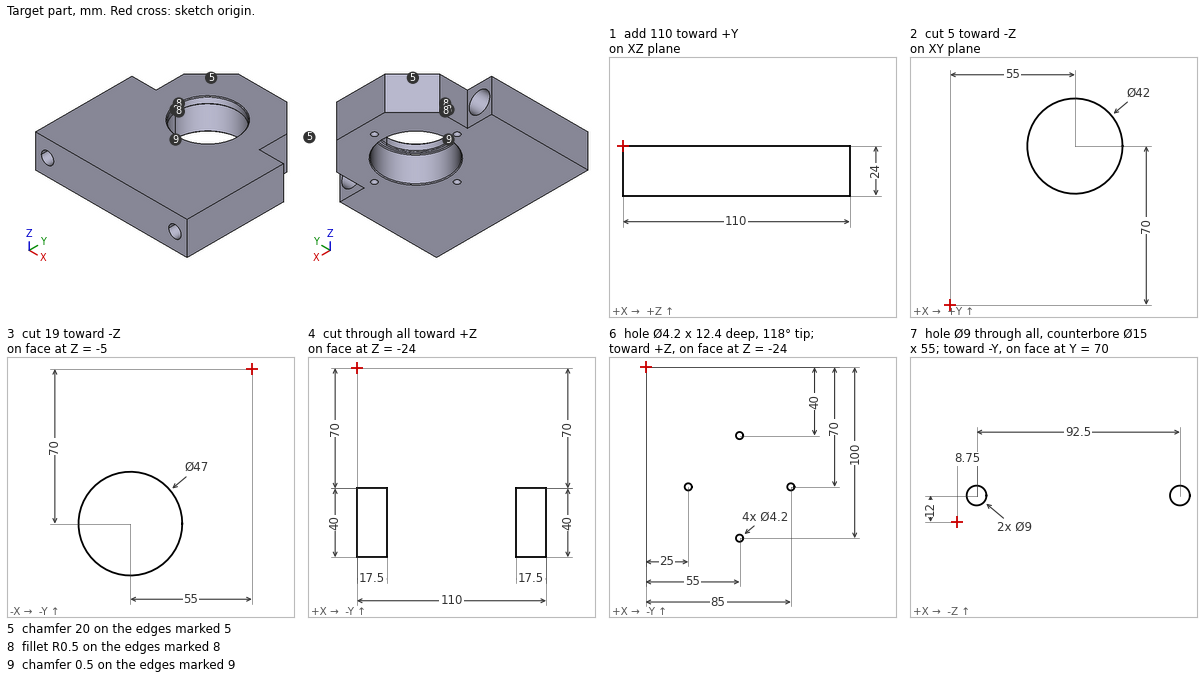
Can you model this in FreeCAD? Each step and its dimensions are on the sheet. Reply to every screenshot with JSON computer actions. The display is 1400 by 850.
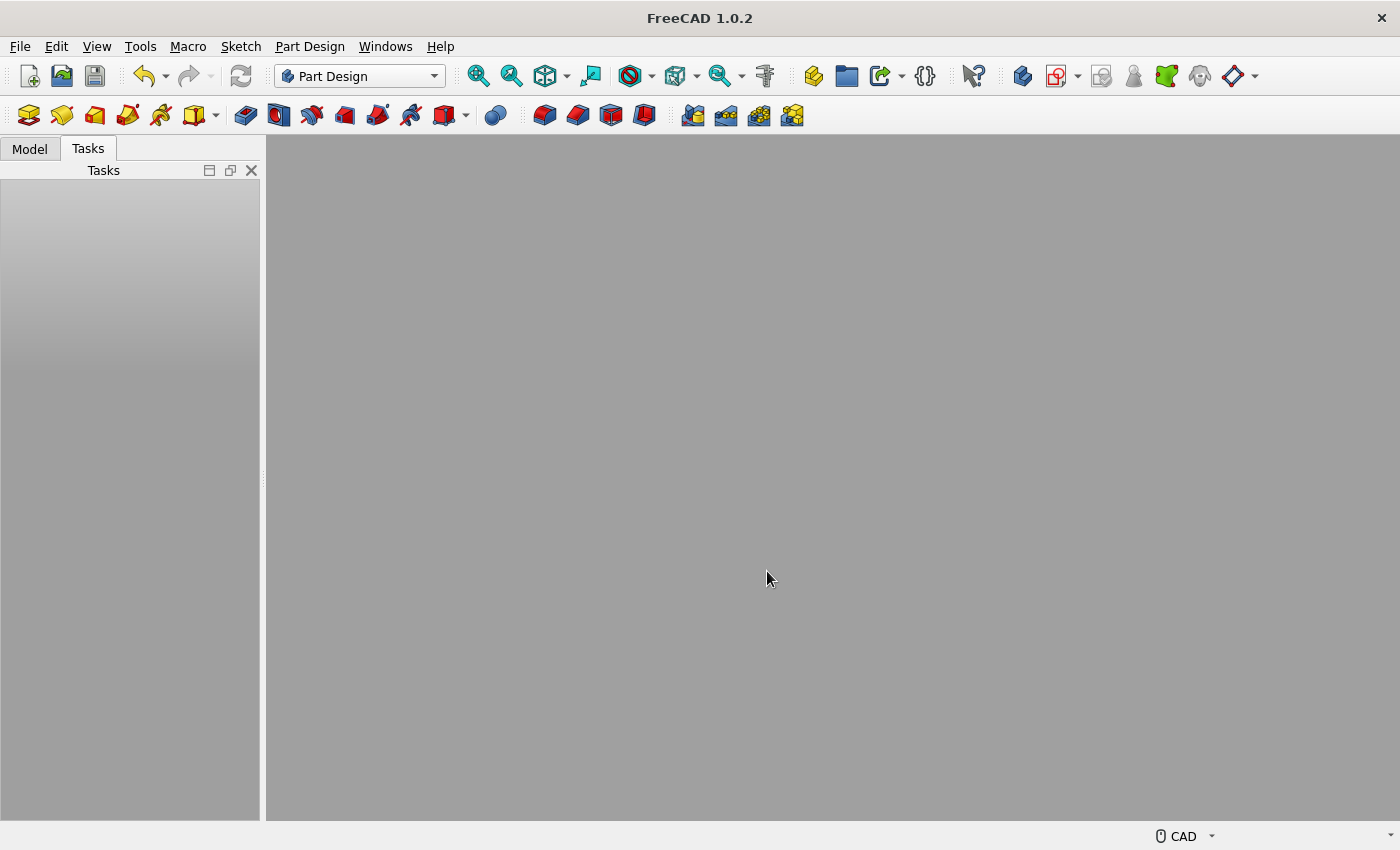
{"action": "left_click", "coordinate": [29, 76]}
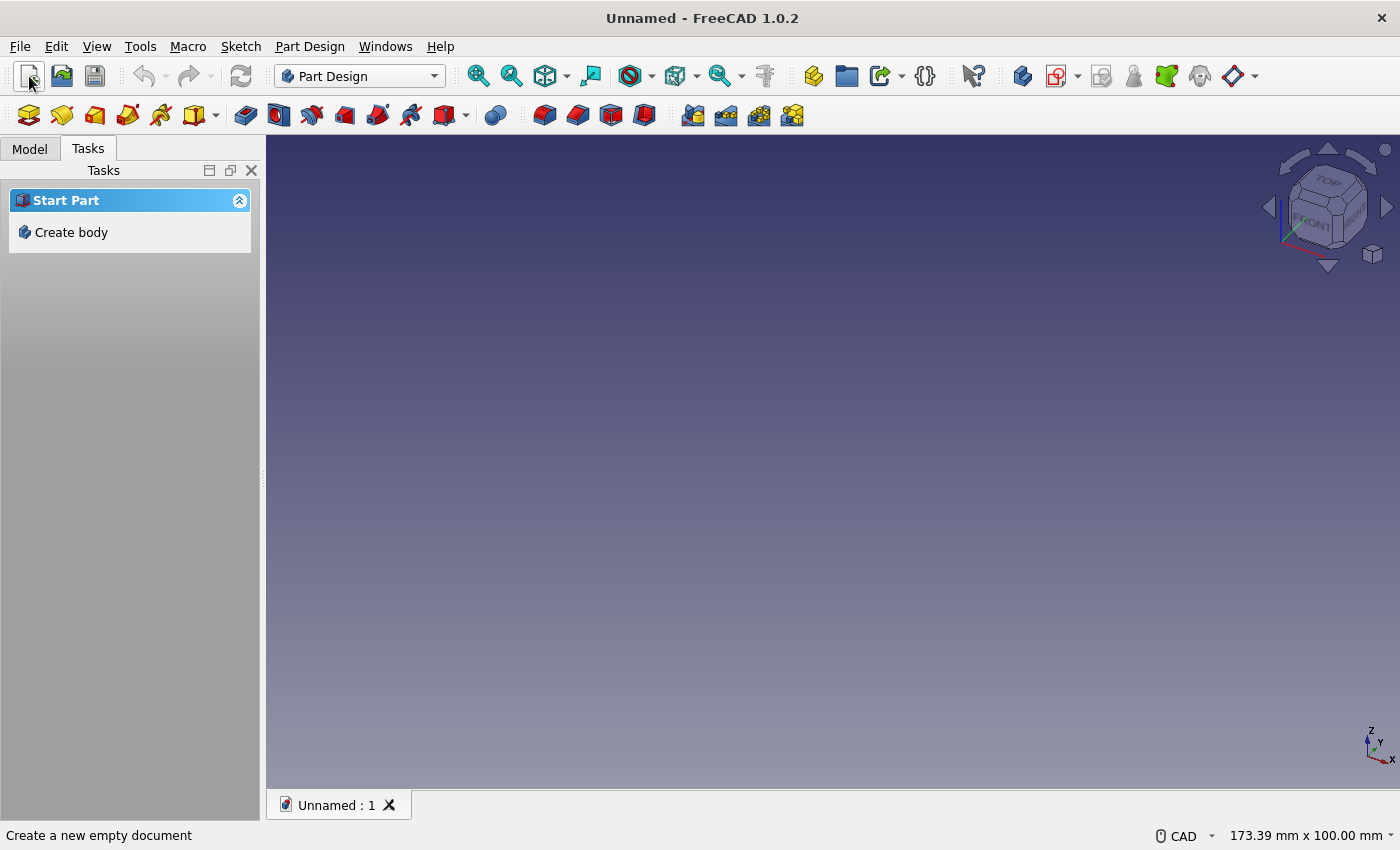
{"action": "left_click", "coordinate": [1056, 76]}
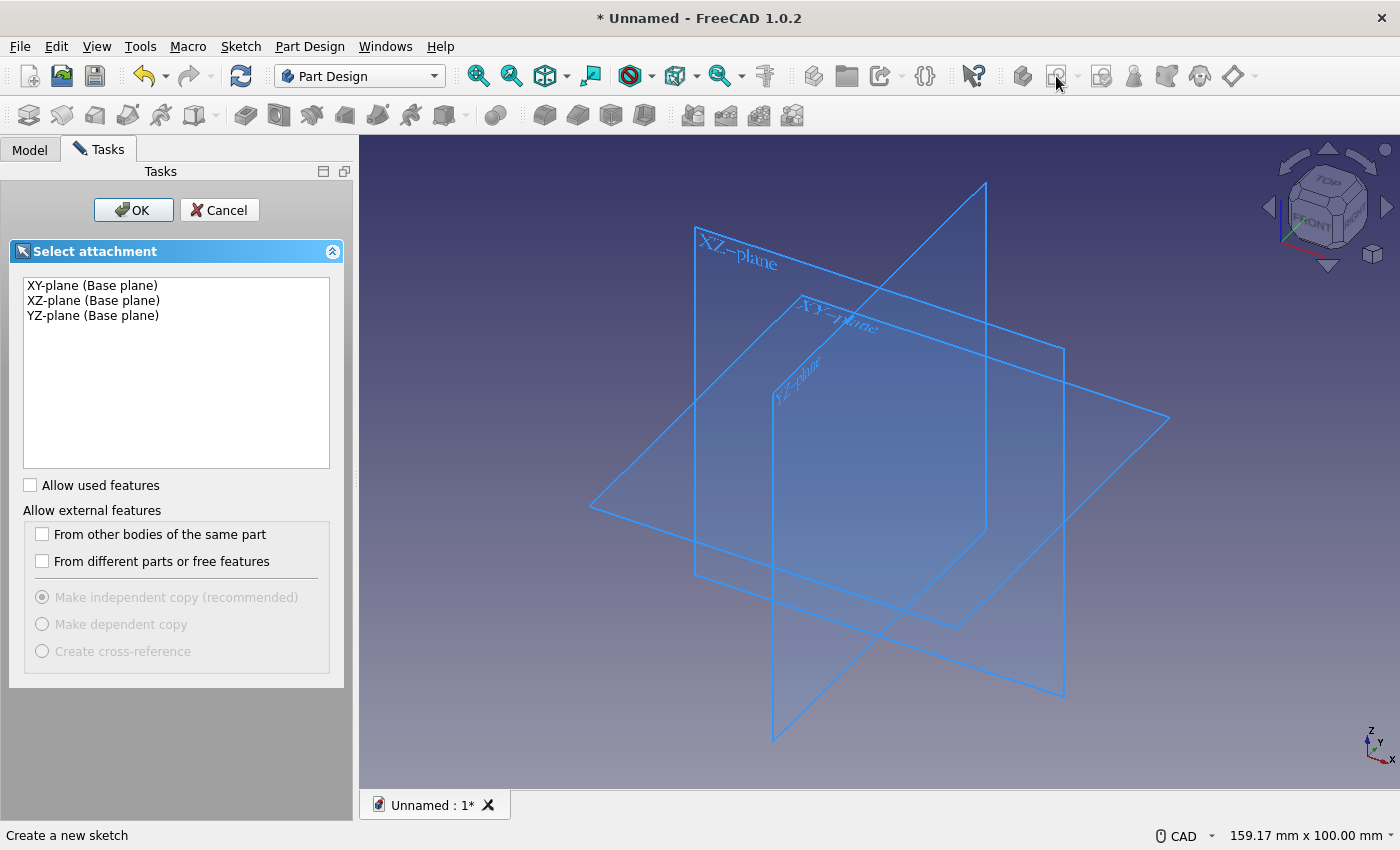
{"action": "left_click", "coordinate": [84, 300]}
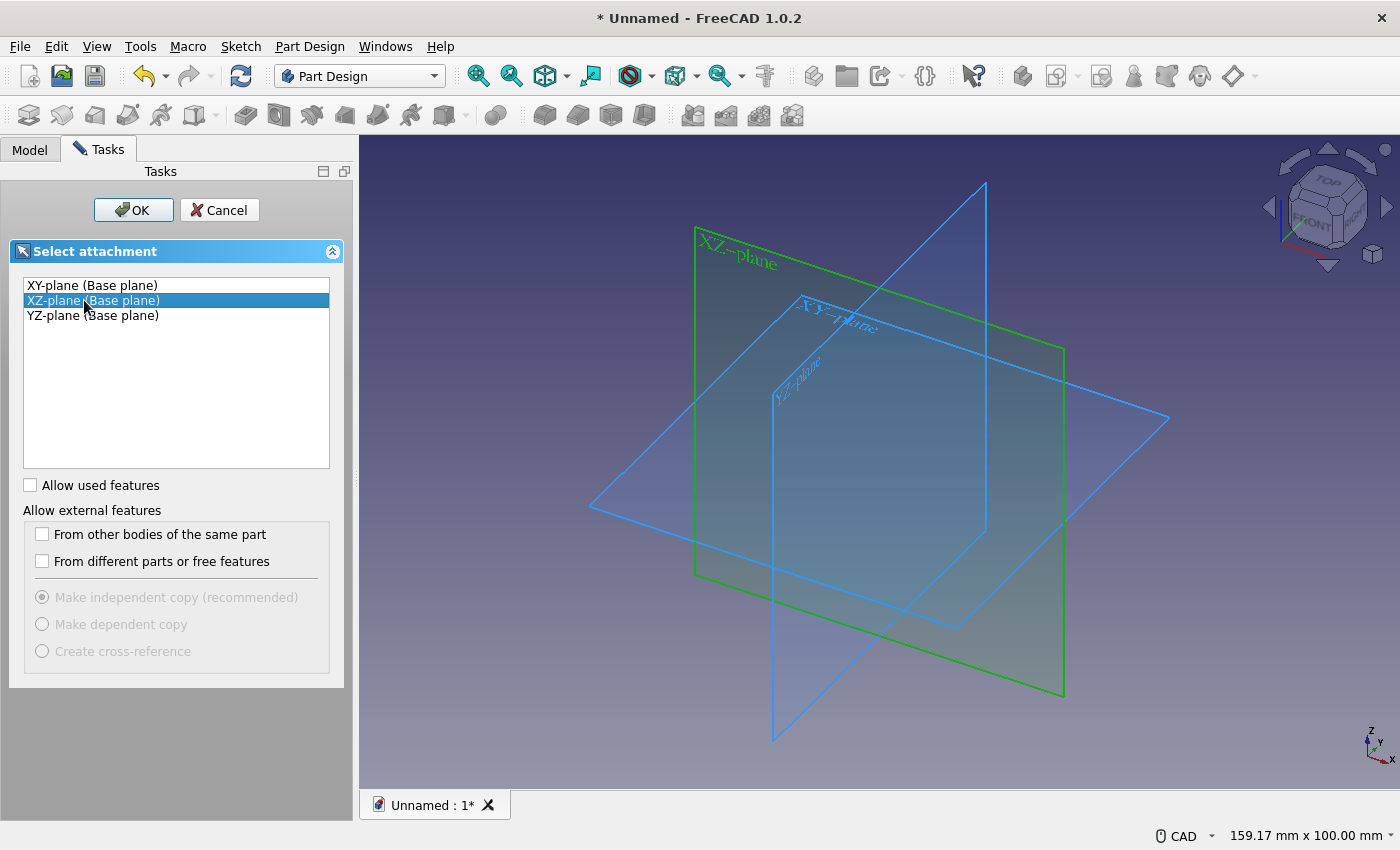
{"action": "left_click", "coordinate": [134, 210]}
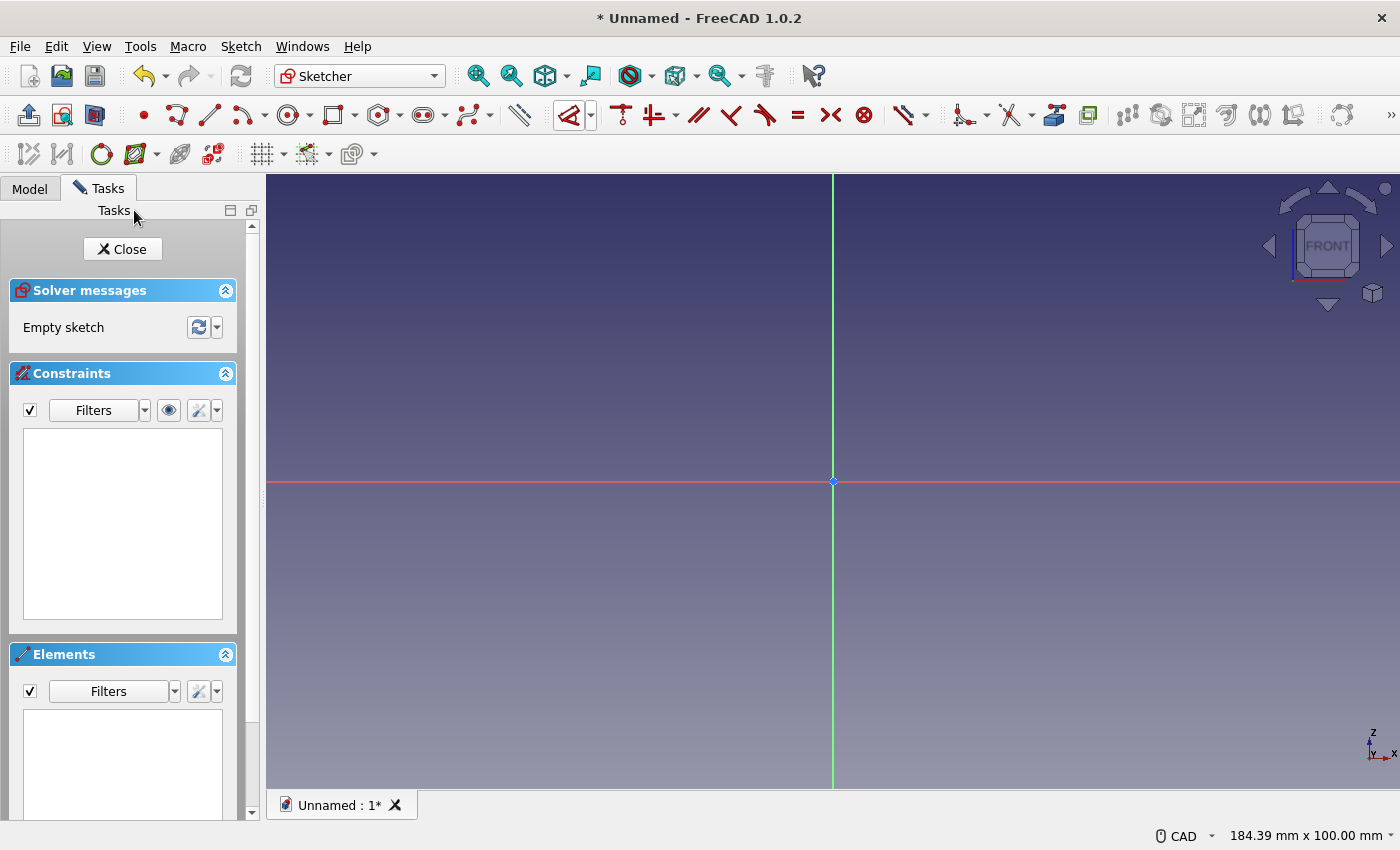
{"action": "scroll", "coordinate": [294, 331], "scroll_direction": "down", "scroll_amount": 2}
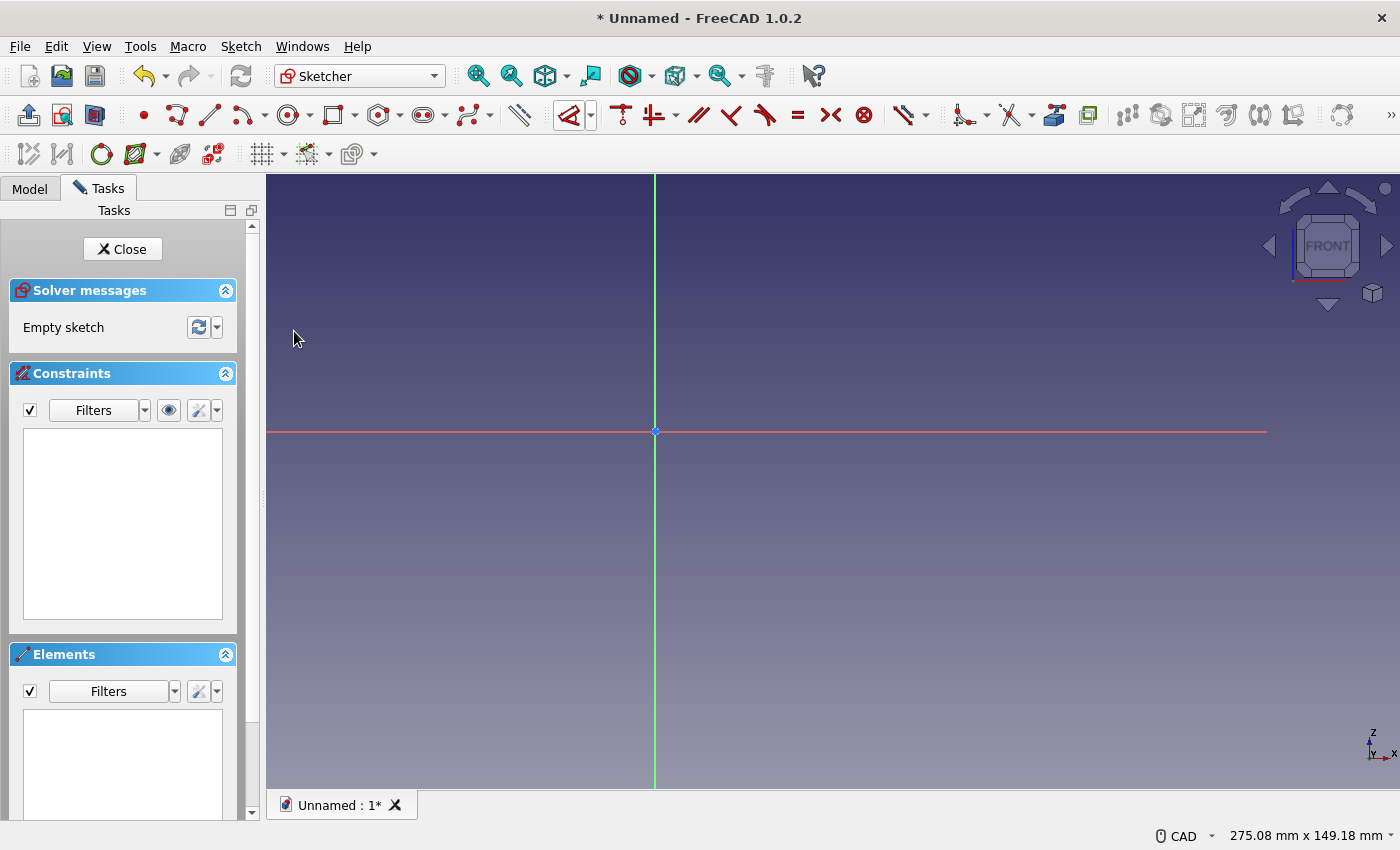
{"action": "scroll", "coordinate": [1121, 481], "scroll_direction": "up", "scroll_amount": 2}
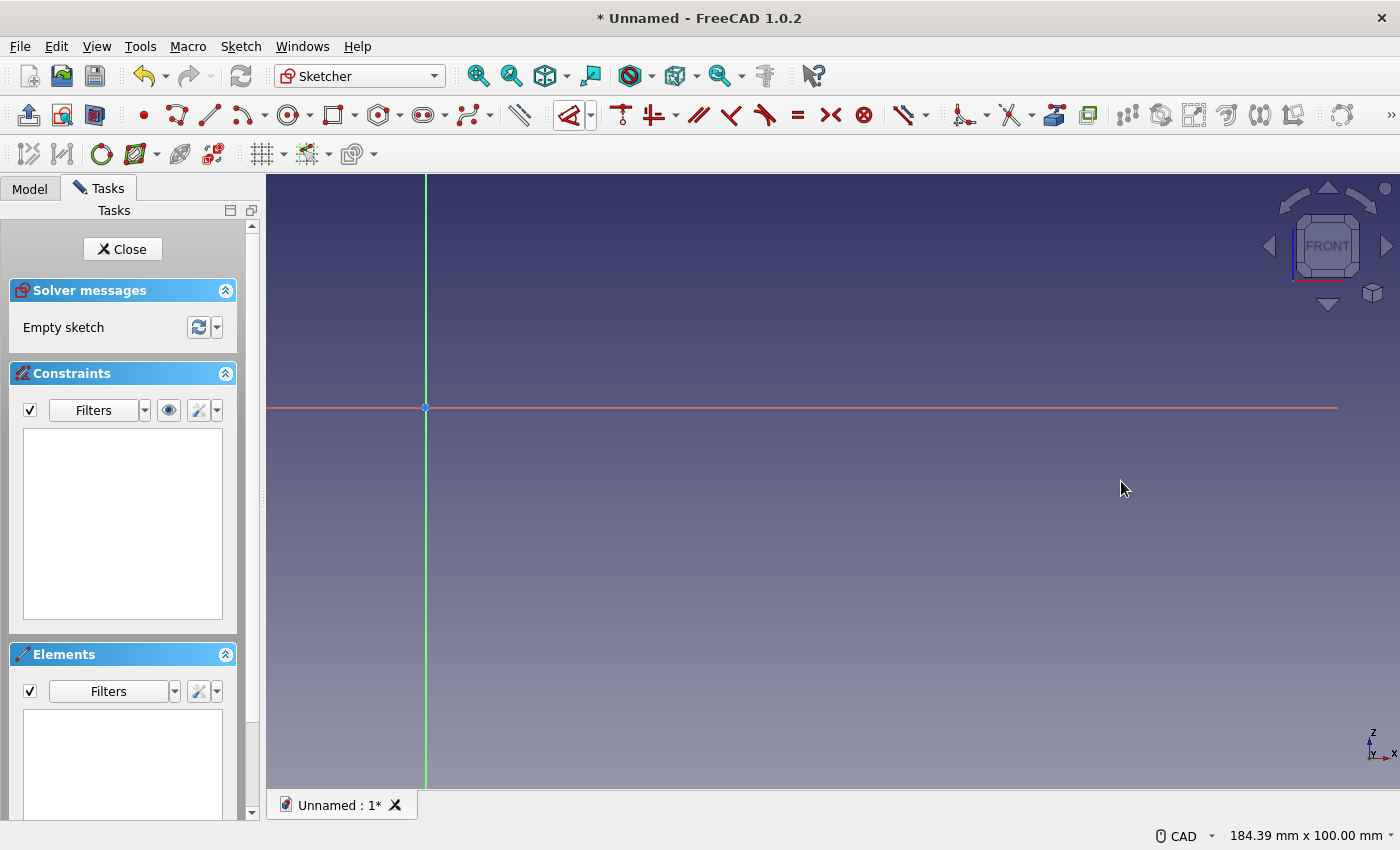
{"action": "left_click", "coordinate": [332, 116]}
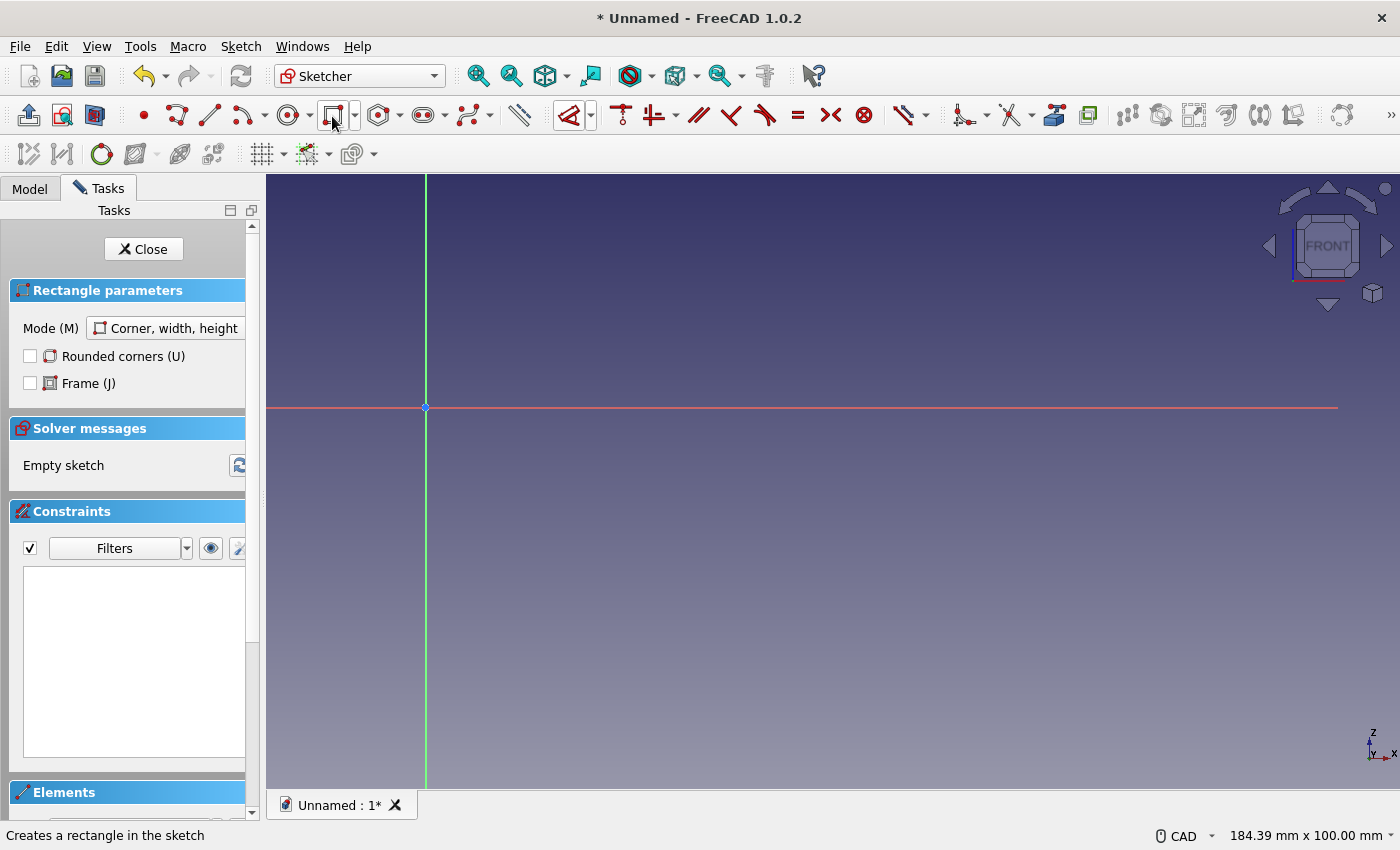
{"action": "left_click", "coordinate": [426, 408]}
{"action": "mouse_move", "coordinate": [1102, 555]}